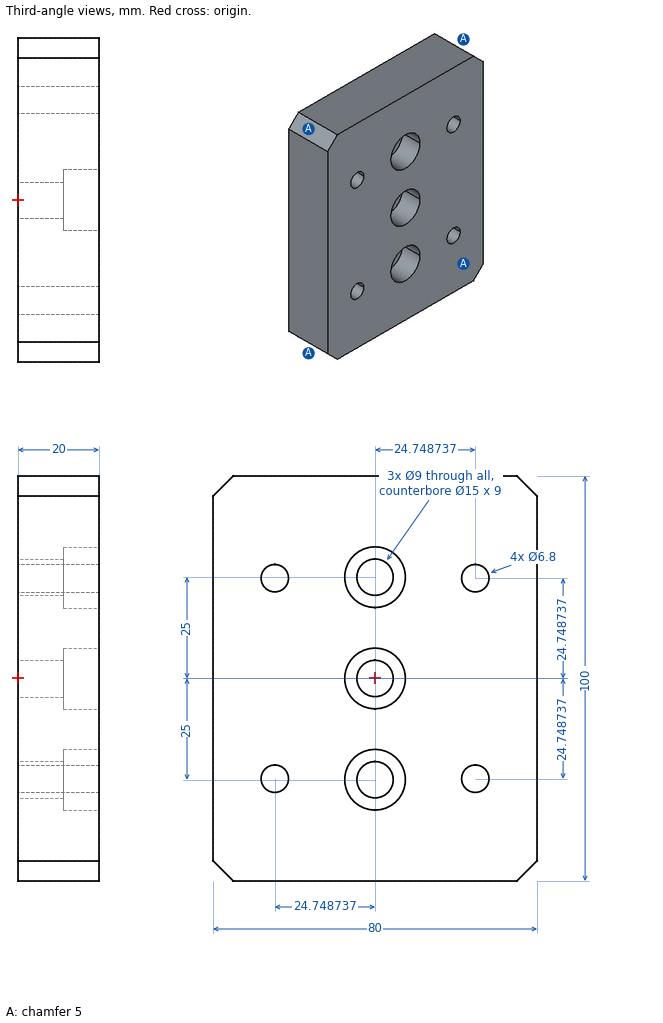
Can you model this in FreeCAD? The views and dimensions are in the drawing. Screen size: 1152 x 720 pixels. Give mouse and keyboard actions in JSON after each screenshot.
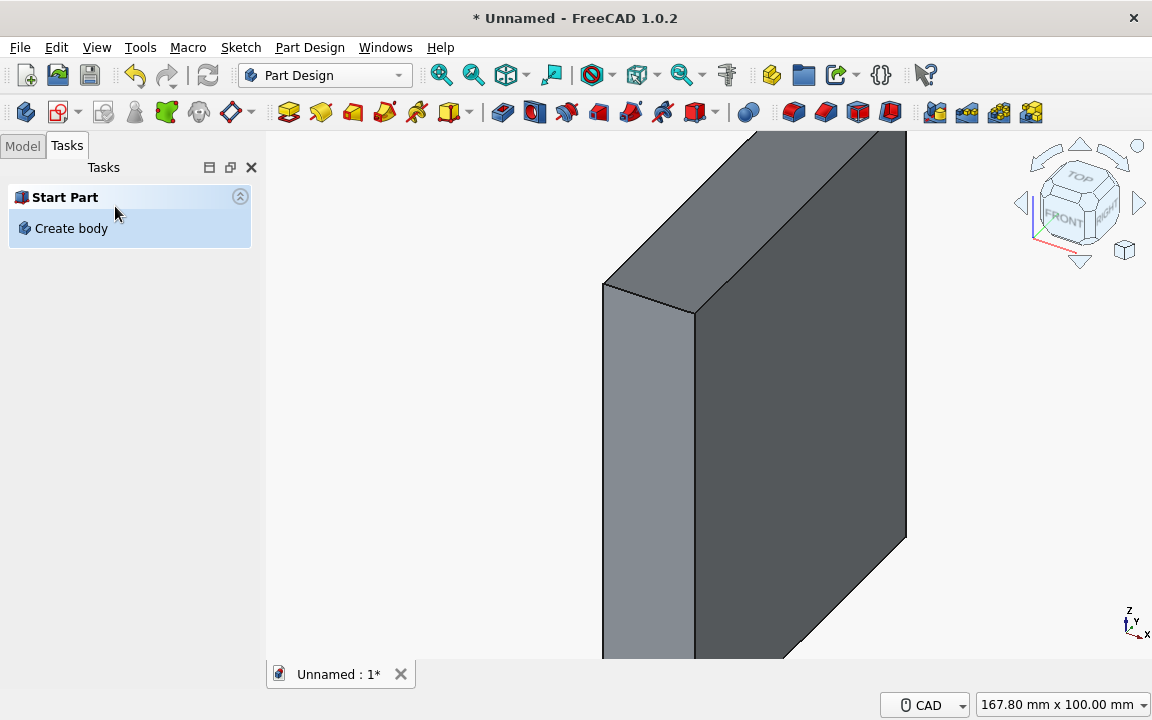
{"action": "key", "text": "v f"}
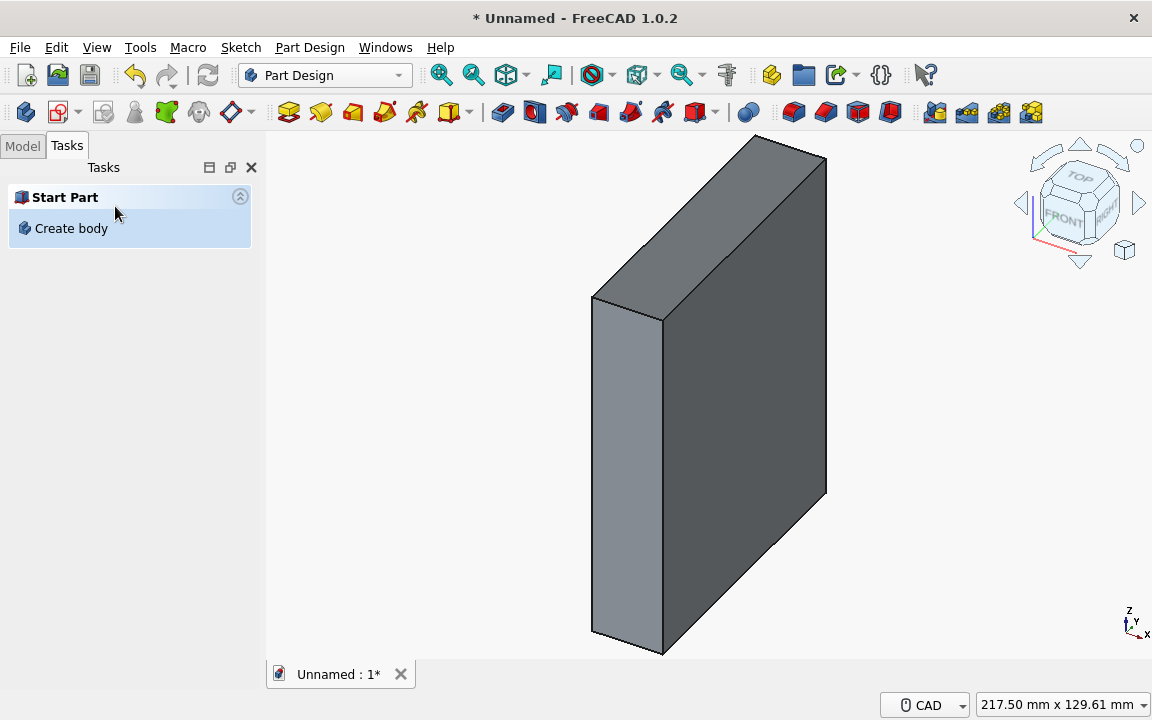
{"action": "left_click", "coordinate": [744, 406]}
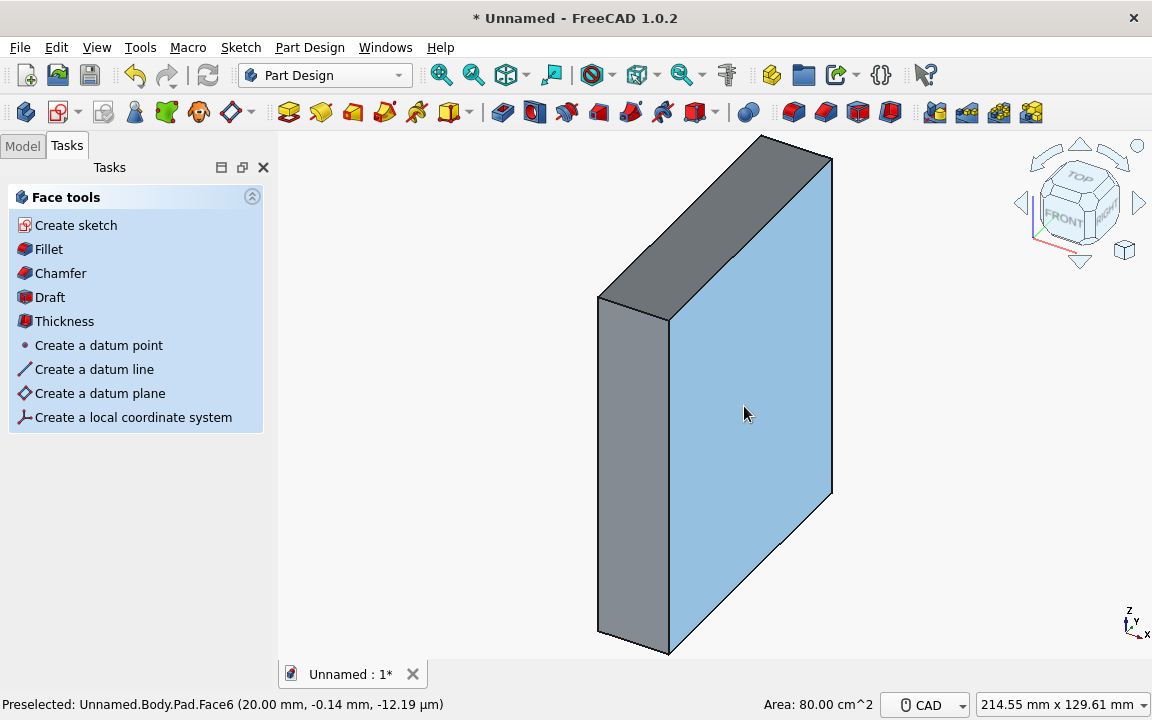
{"action": "left_click", "coordinate": [58, 112]}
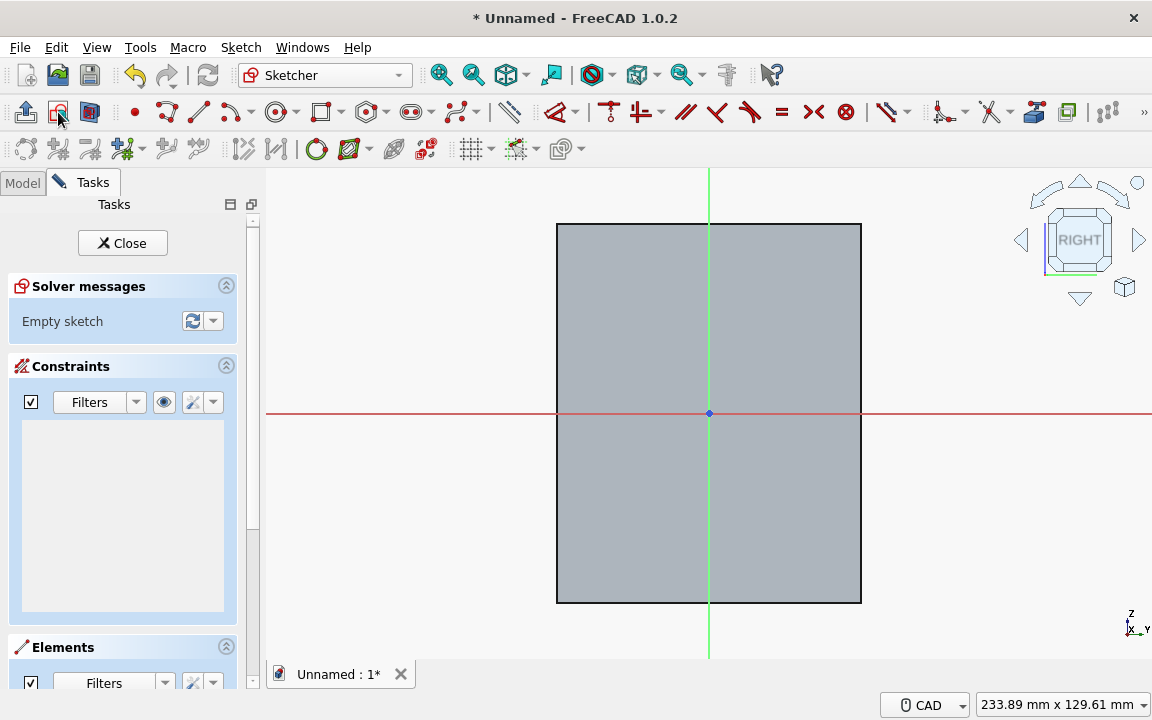
{"action": "scroll", "coordinate": [848, 413], "scroll_direction": "up", "scroll_amount": 2}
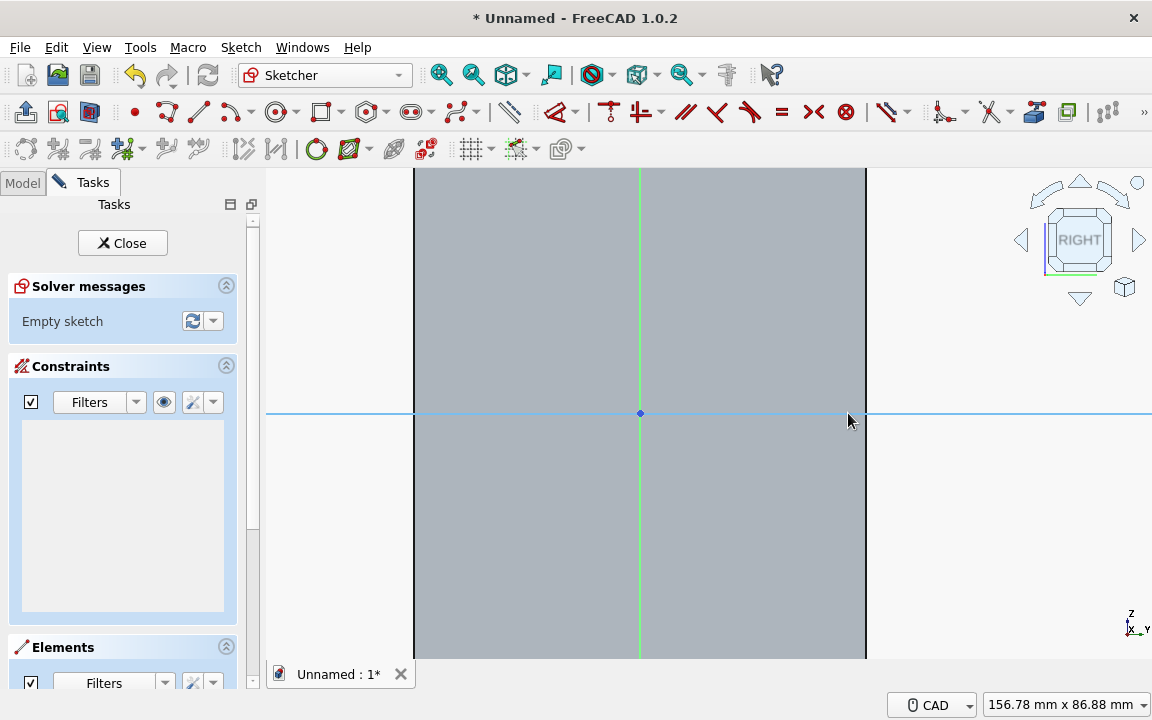
{"action": "key", "text": "g c"}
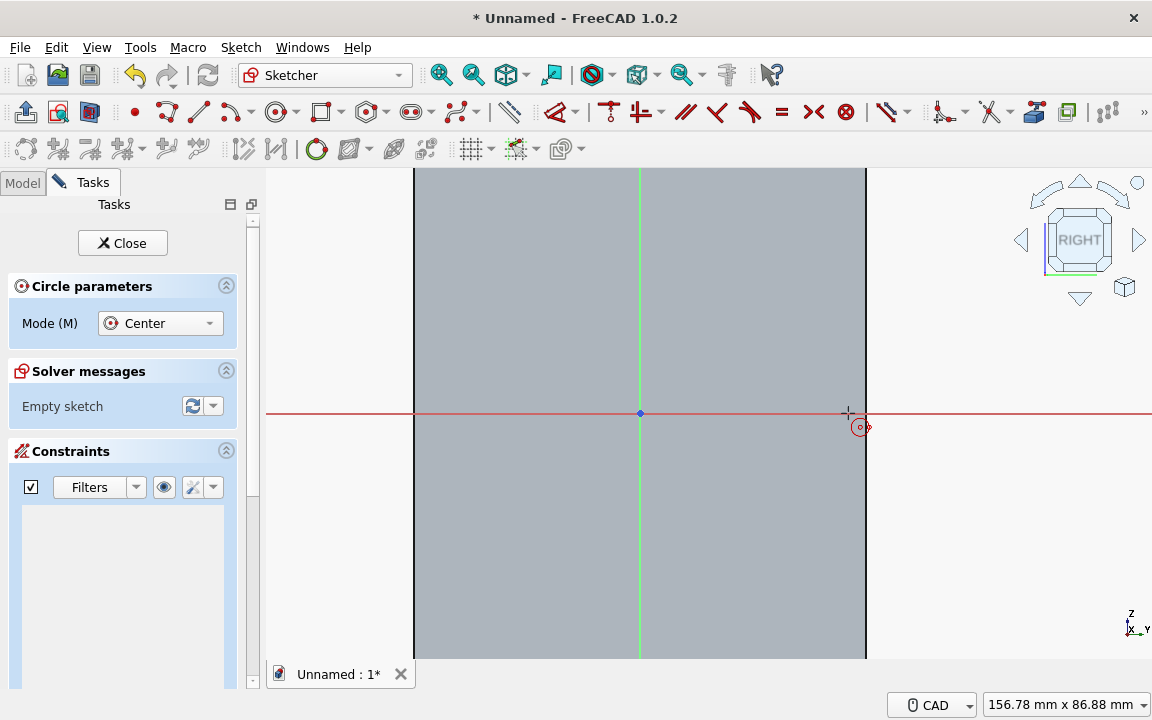
{"action": "left_click", "coordinate": [780, 274]}
{"action": "mouse_move", "coordinate": [794, 260]}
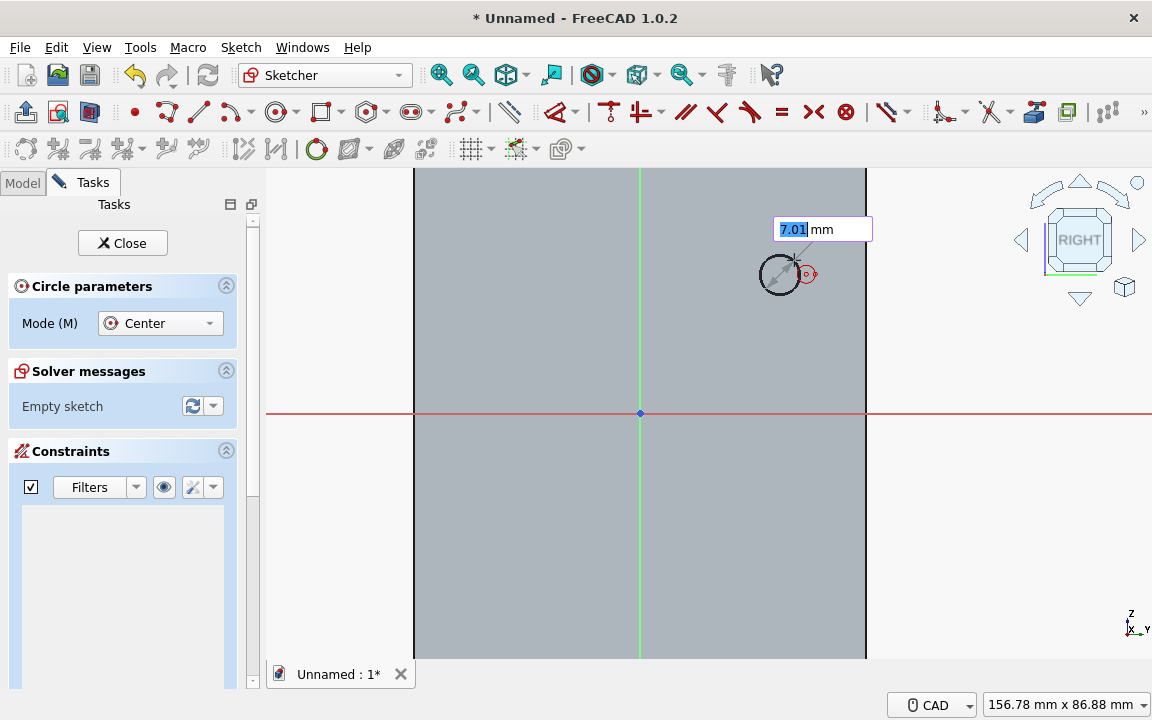
{"action": "type", "text": "6.8"}
{"action": "key", "text": "Return"}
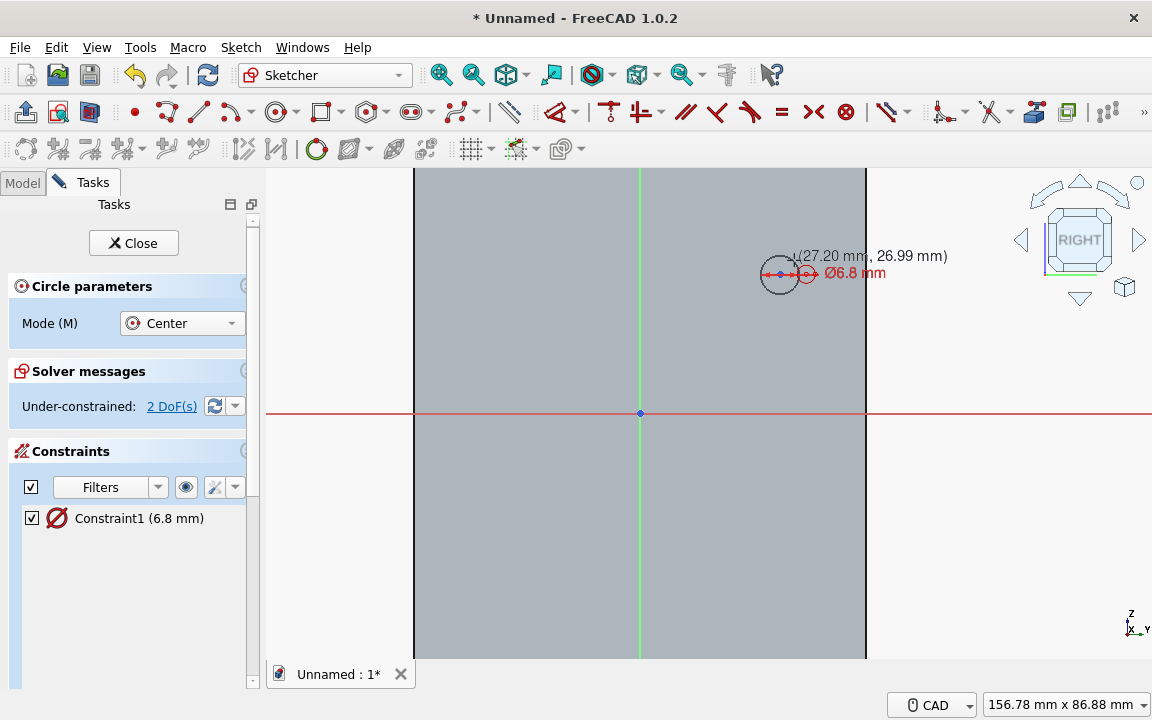
{"action": "left_click", "coordinate": [780, 553]}
{"action": "mouse_move", "coordinate": [794, 540]}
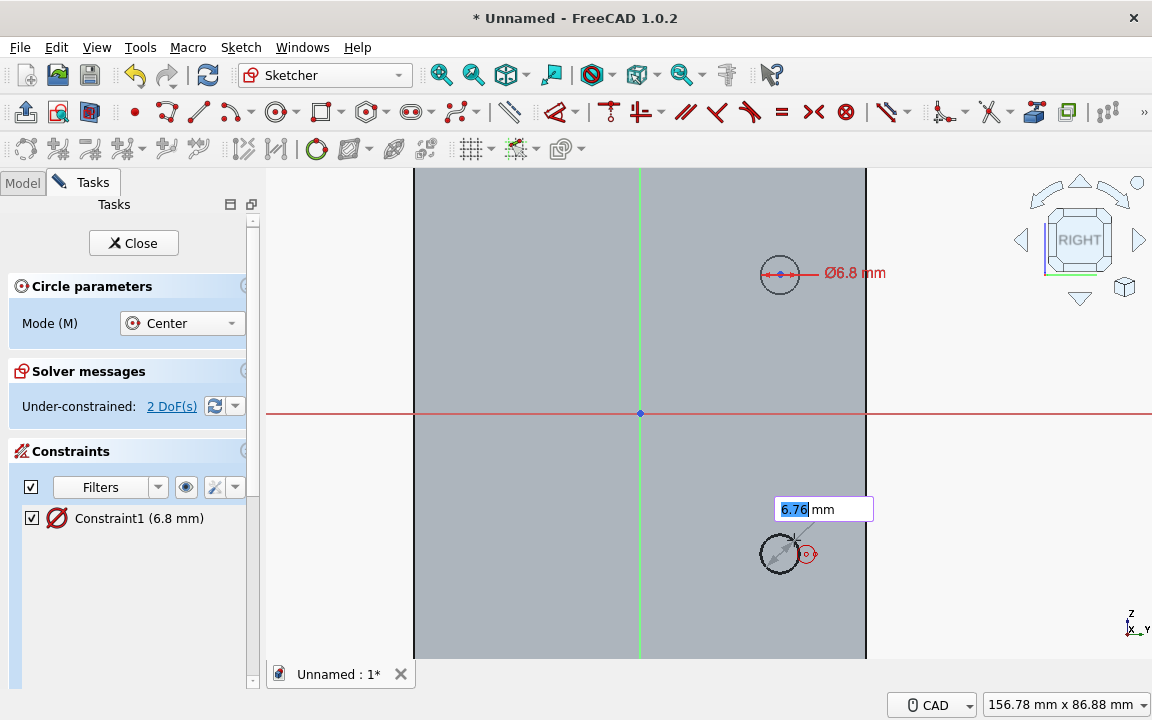
{"action": "type", "text": "6.8"}
{"action": "key", "text": "Return"}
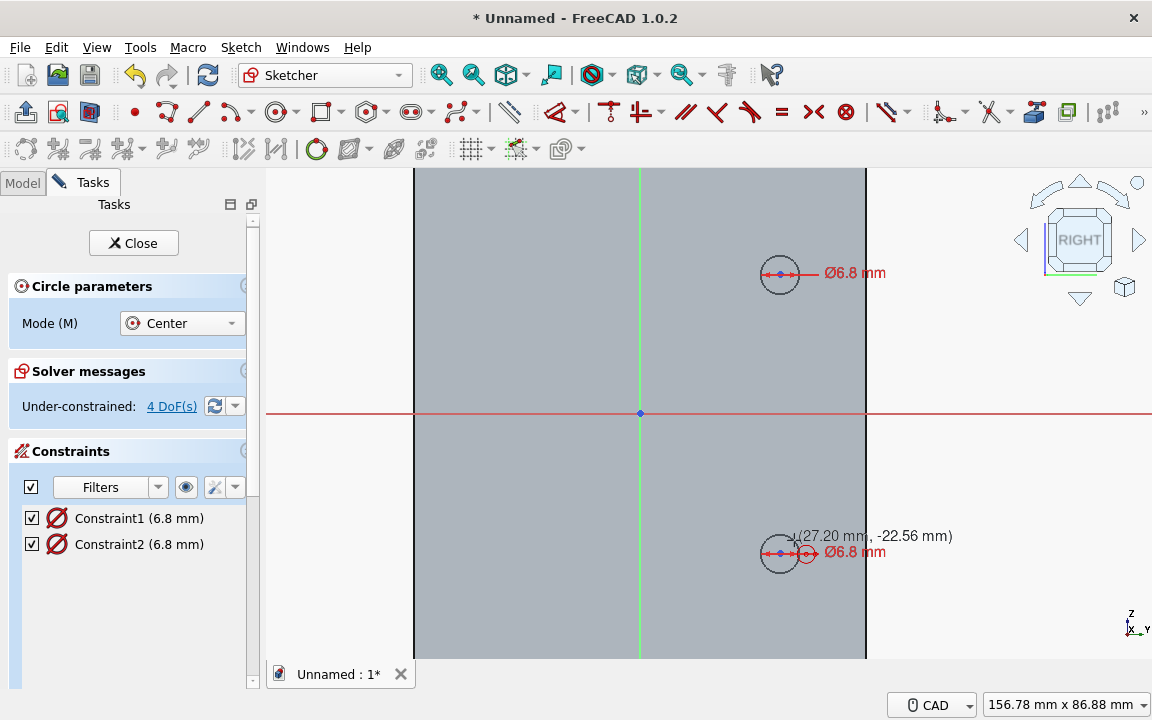
{"action": "left_click", "coordinate": [500, 553]}
{"action": "mouse_move", "coordinate": [514, 540]}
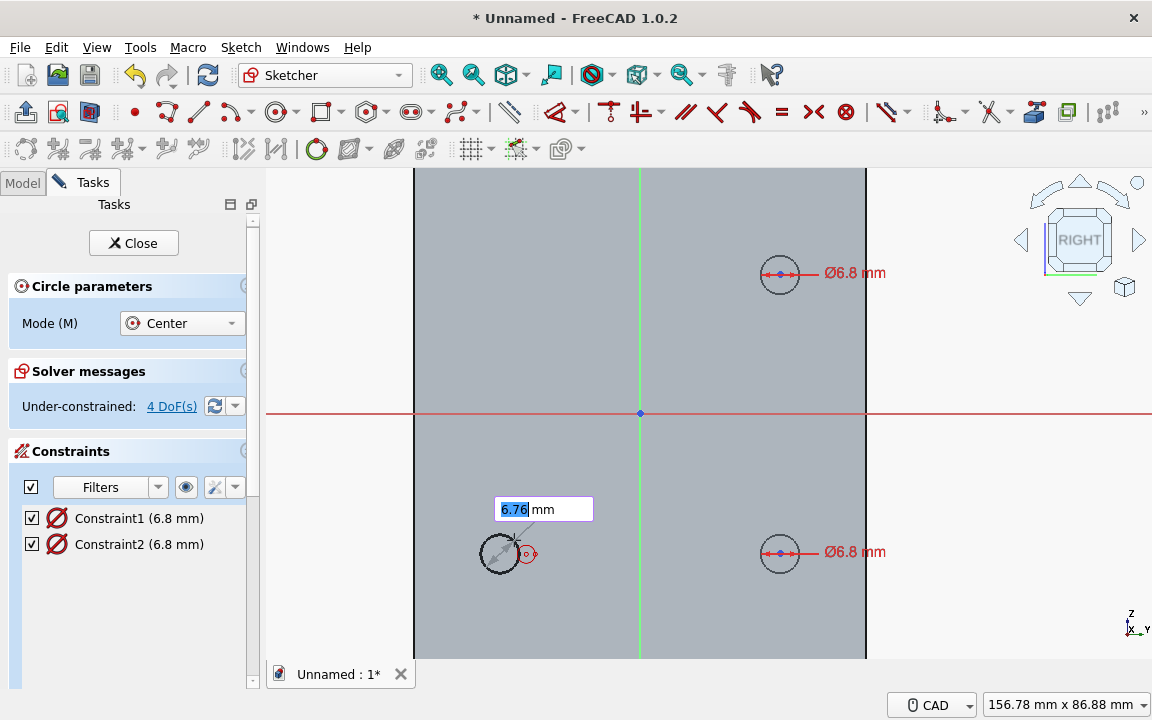
{"action": "type", "text": "6.8"}
{"action": "key", "text": "Return"}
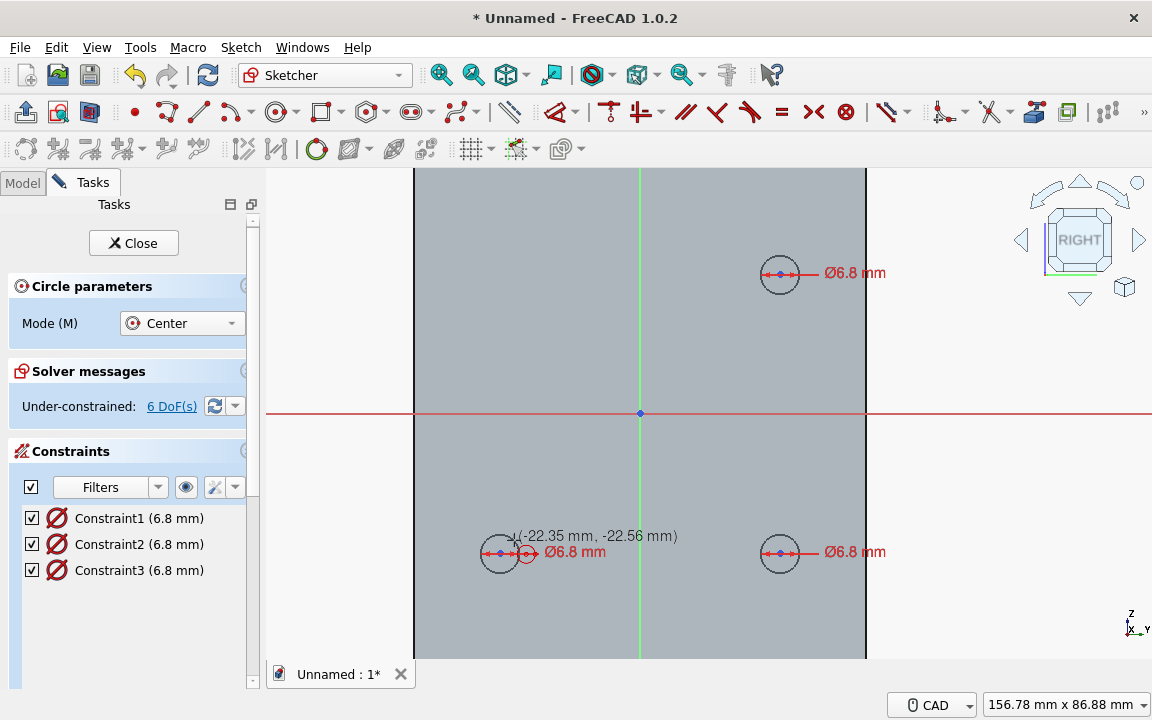
{"action": "left_click", "coordinate": [500, 274]}
{"action": "mouse_move", "coordinate": [514, 260]}